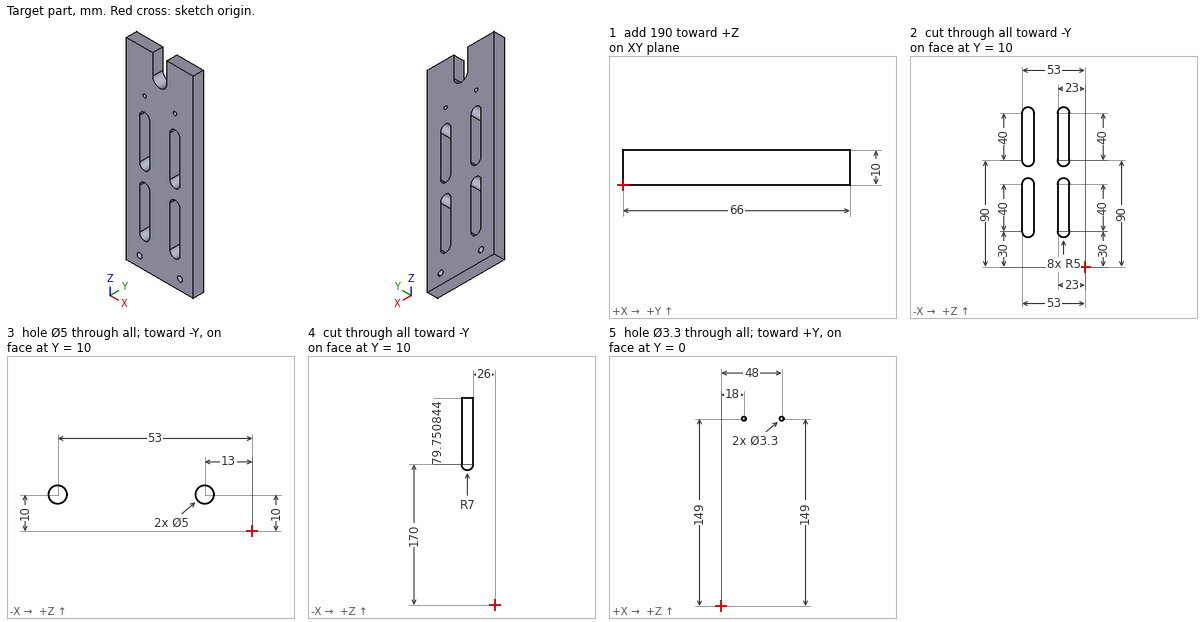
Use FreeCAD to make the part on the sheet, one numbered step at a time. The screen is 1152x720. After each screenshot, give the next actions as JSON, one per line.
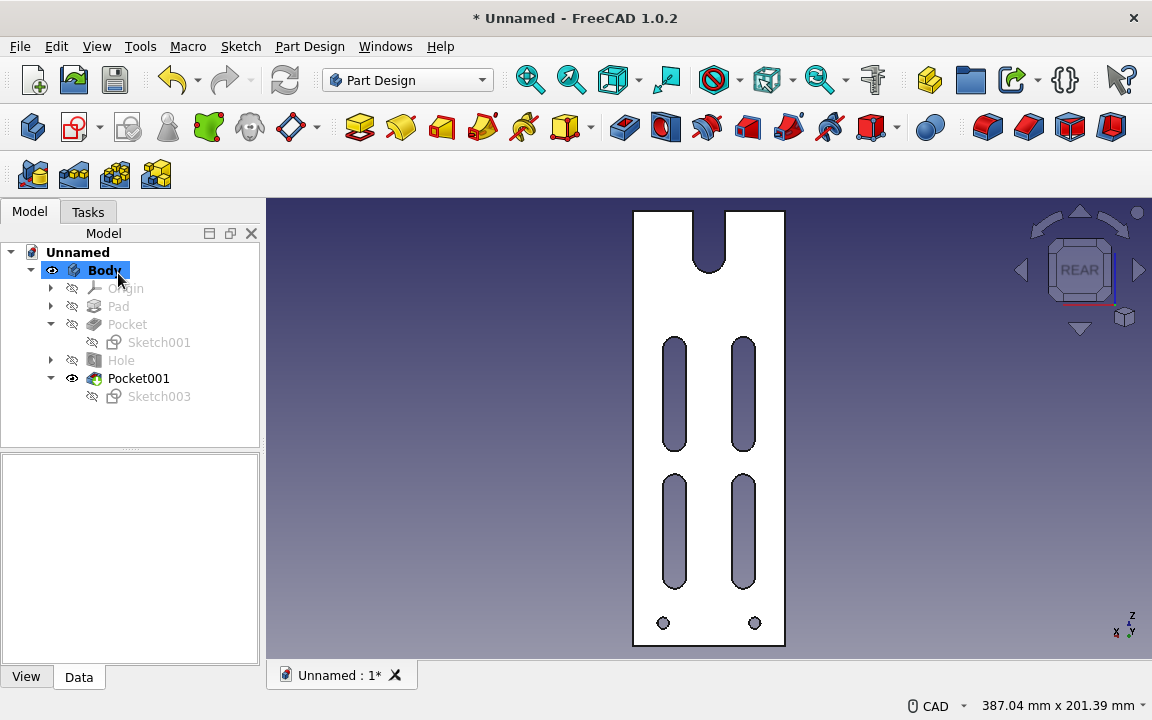
{"action": "key", "text": "0"}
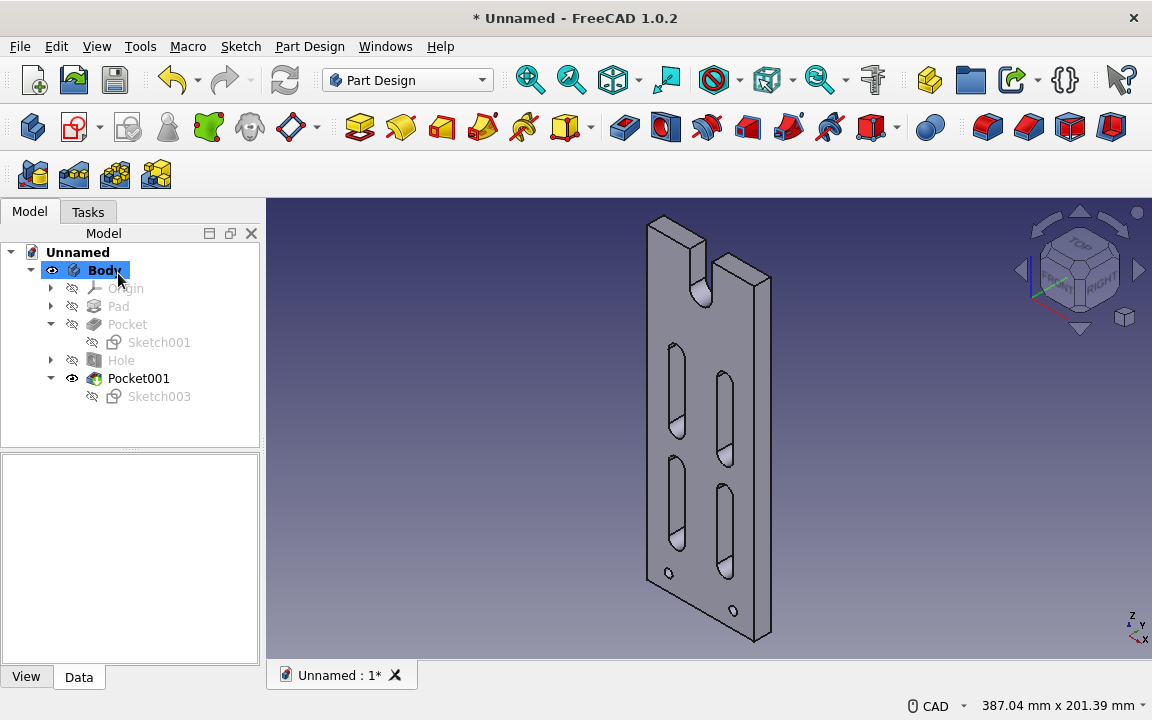
{"action": "left_click", "coordinate": [716, 340]}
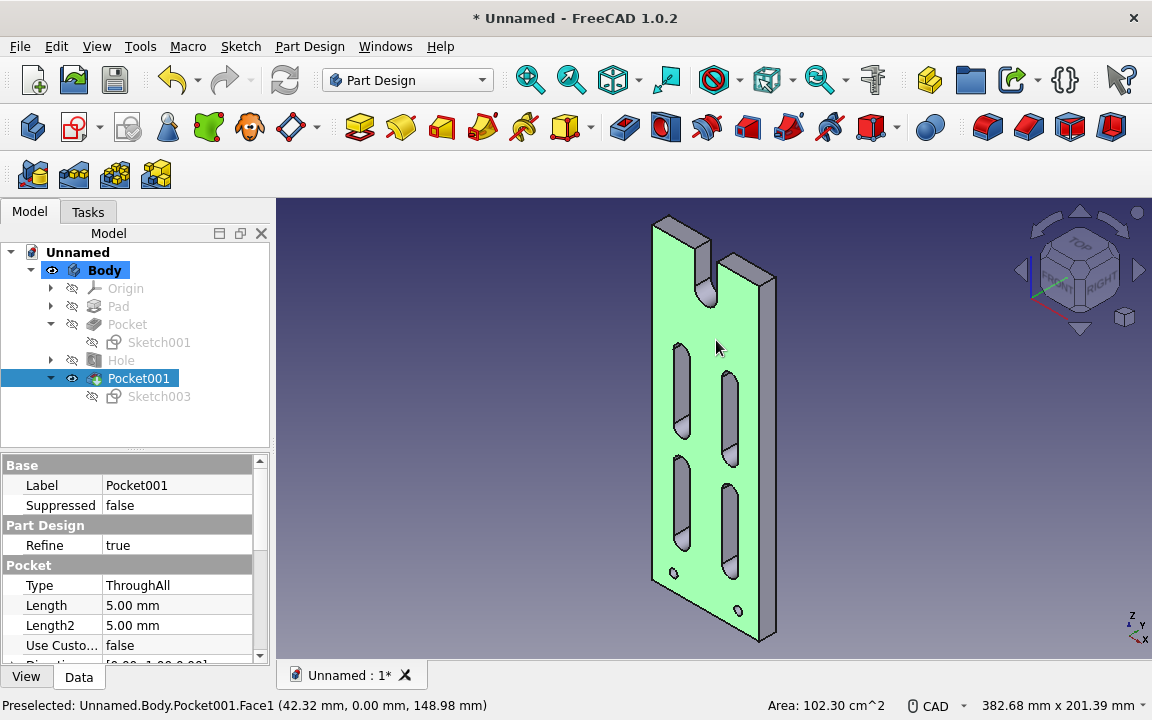
{"action": "left_click", "coordinate": [74, 128]}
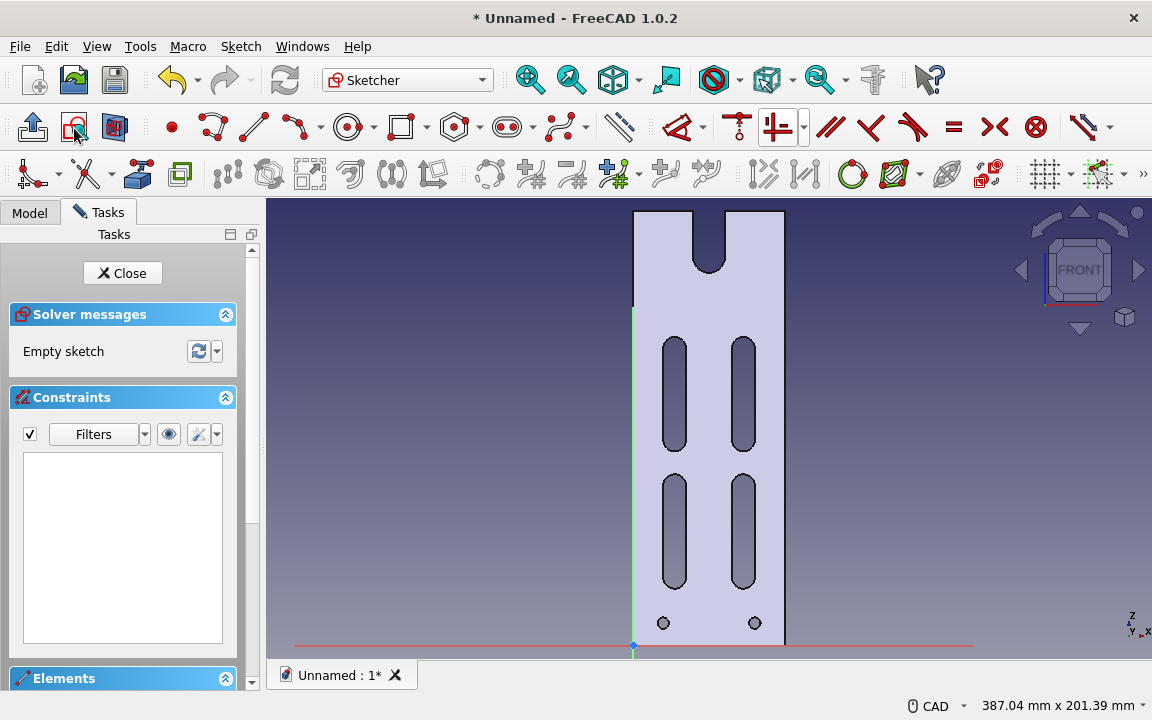
{"action": "scroll", "coordinate": [723, 280], "scroll_direction": "up", "scroll_amount": 9}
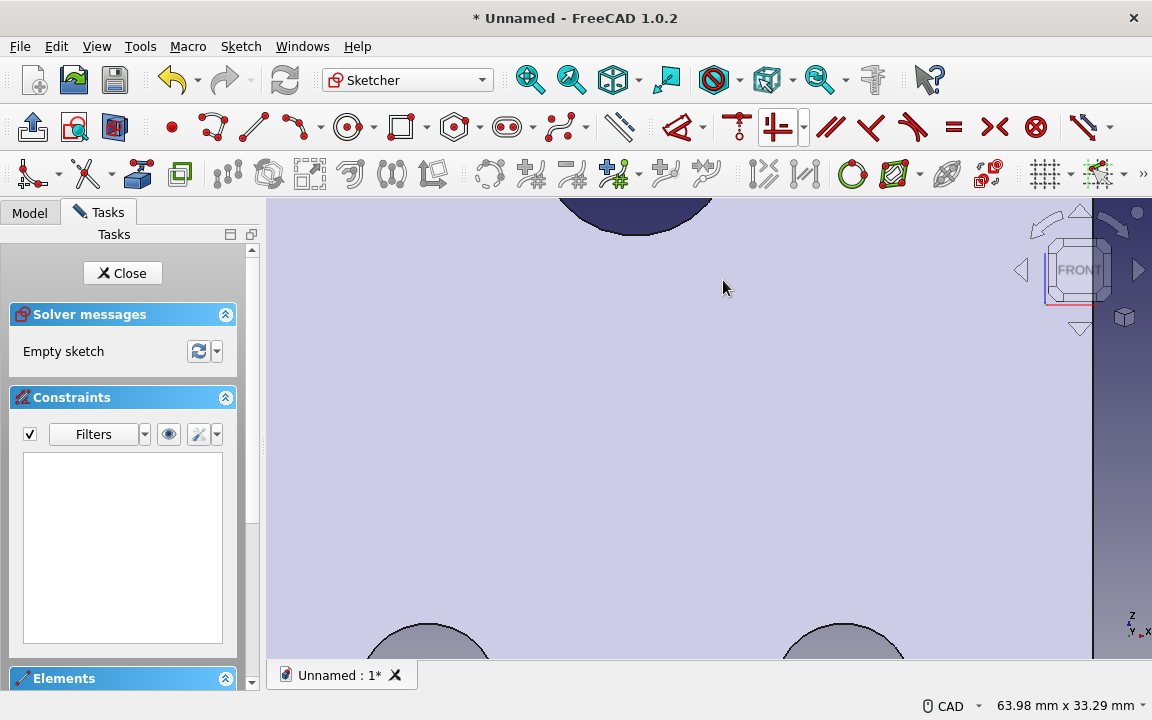
{"action": "left_click", "coordinate": [348, 128]}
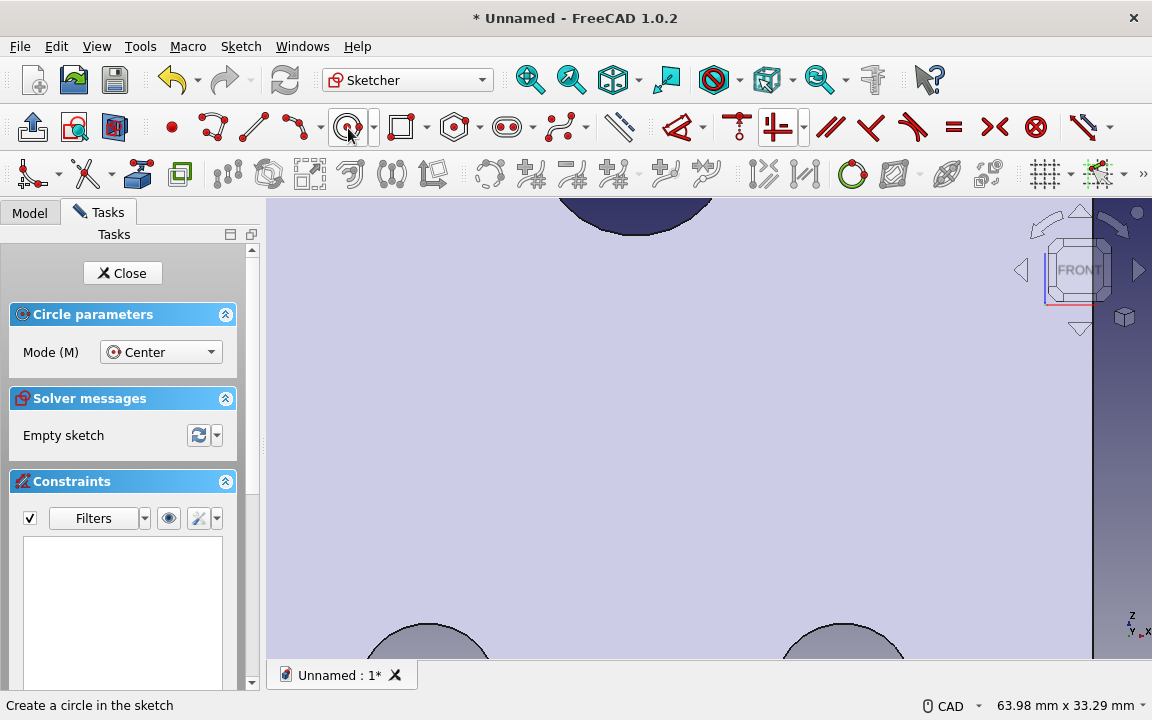
{"action": "left_click", "coordinate": [428, 430]}
{"action": "mouse_move", "coordinate": [444, 413]}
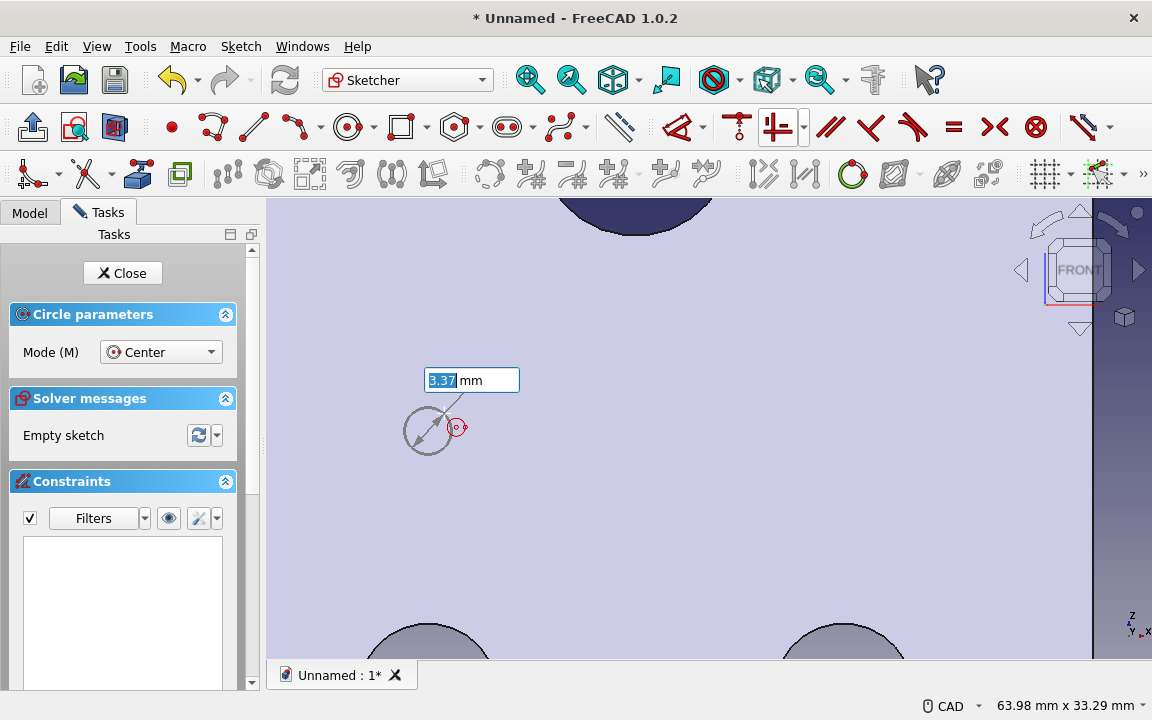
{"action": "type", "text": "3.3"}
{"action": "key", "text": "Return"}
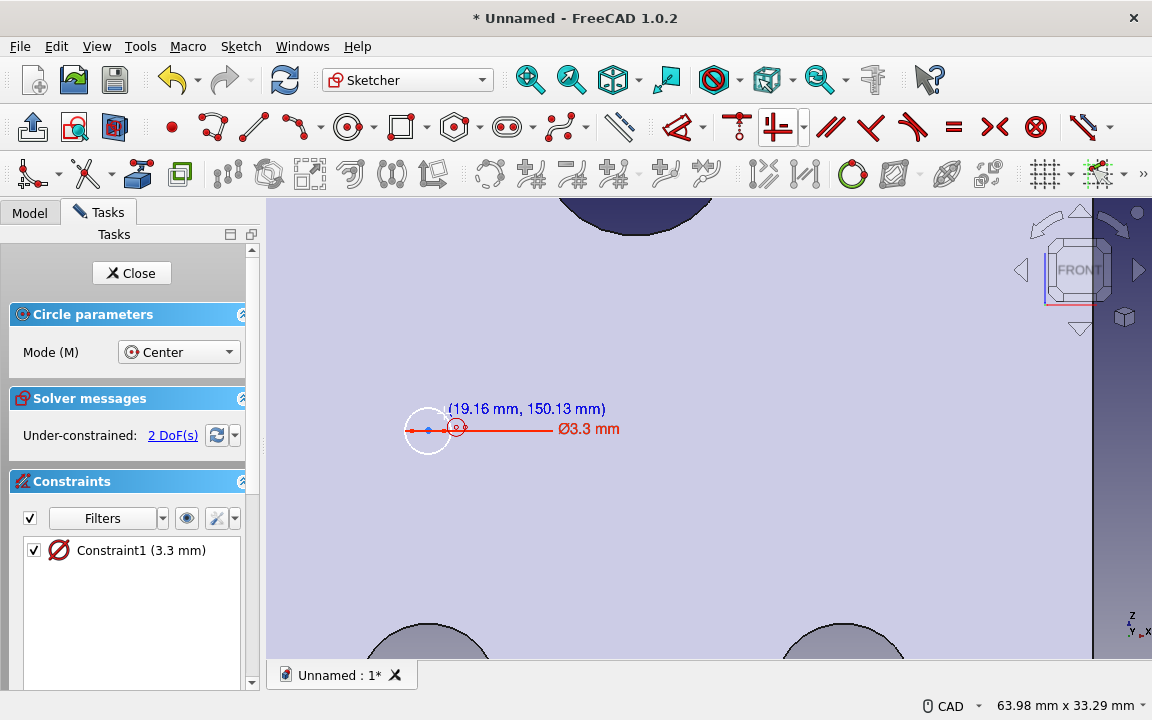
{"action": "left_click", "coordinate": [843, 430]}
{"action": "mouse_move", "coordinate": [860, 413]}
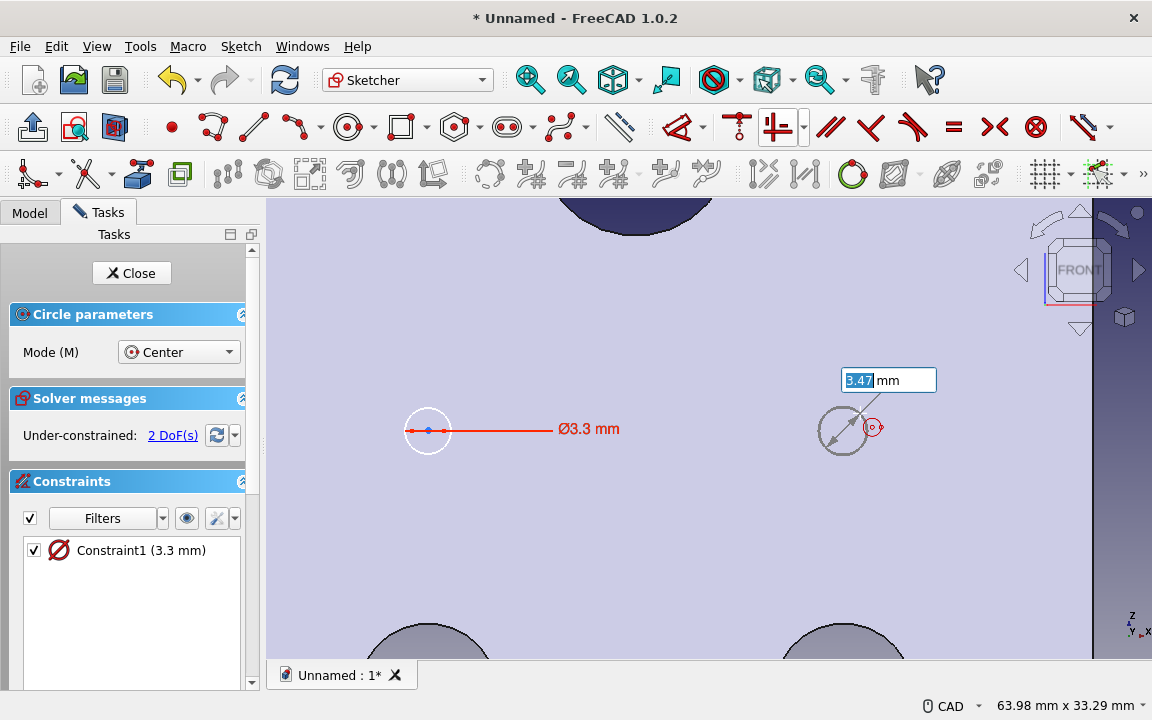
{"action": "type", "text": "3.3"}
{"action": "key", "text": "Return"}
{"action": "key", "text": "Escape"}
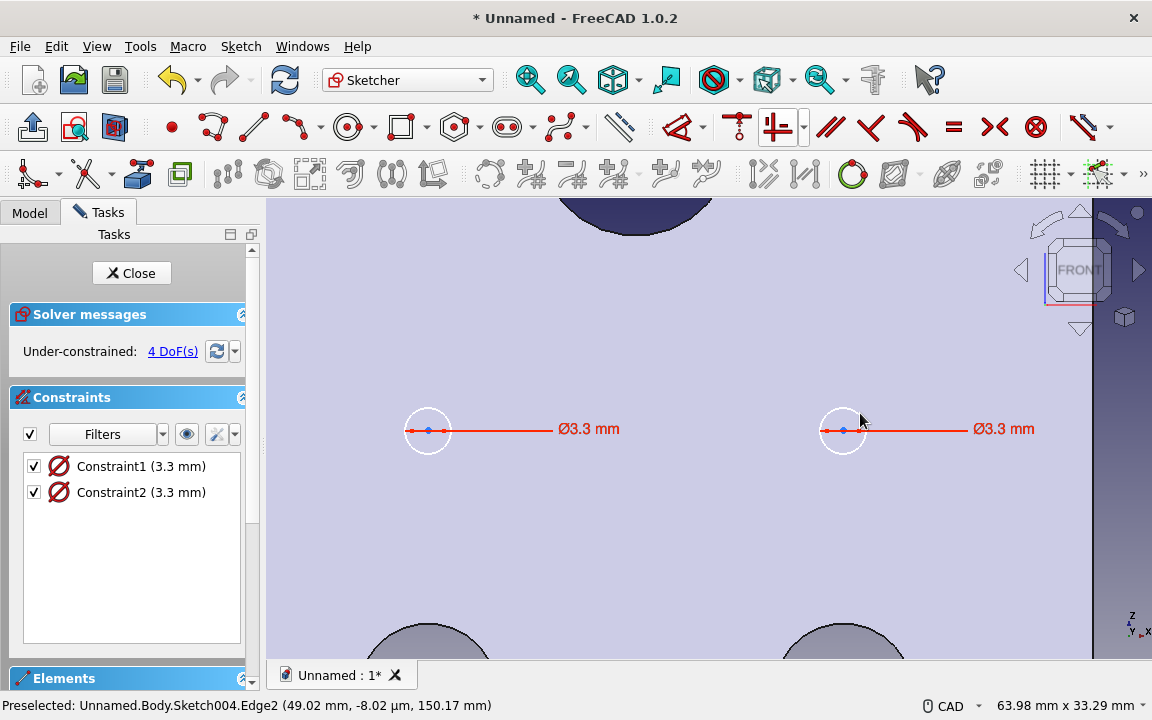
{"action": "left_click", "coordinate": [676, 128]}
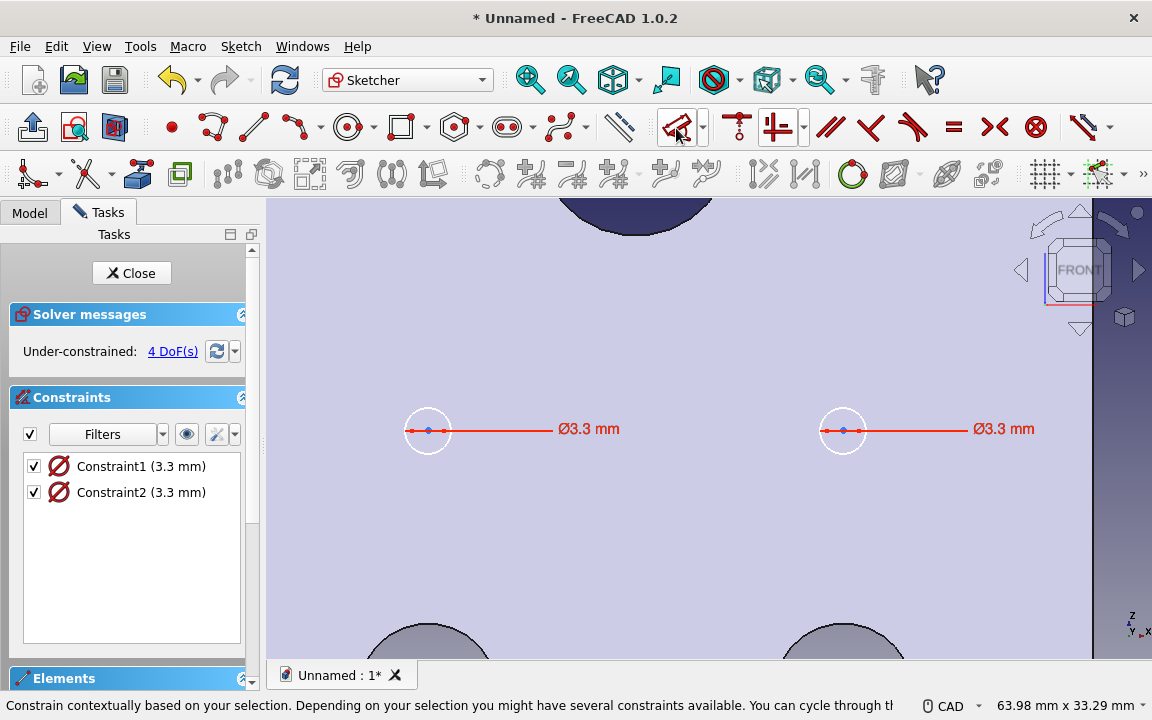
{"action": "left_click", "coordinate": [428, 431]}
{"action": "left_click", "coordinate": [361, 397]}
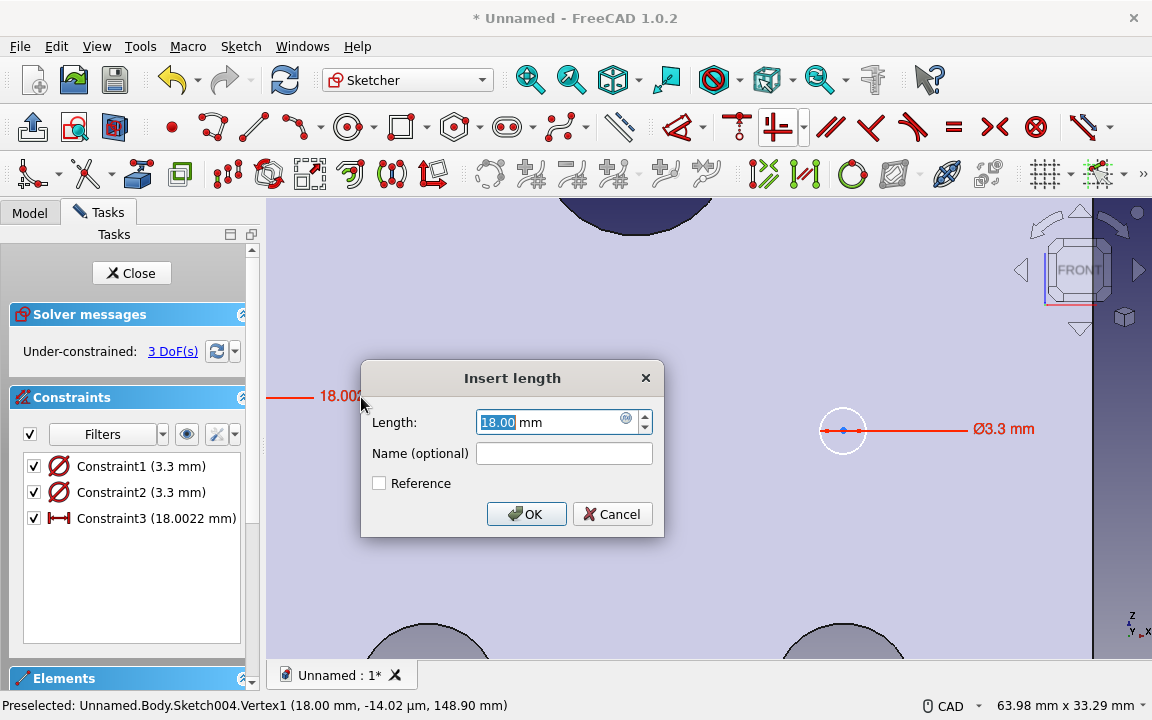
{"action": "type", "text": "18"}
{"action": "key", "text": "Return"}